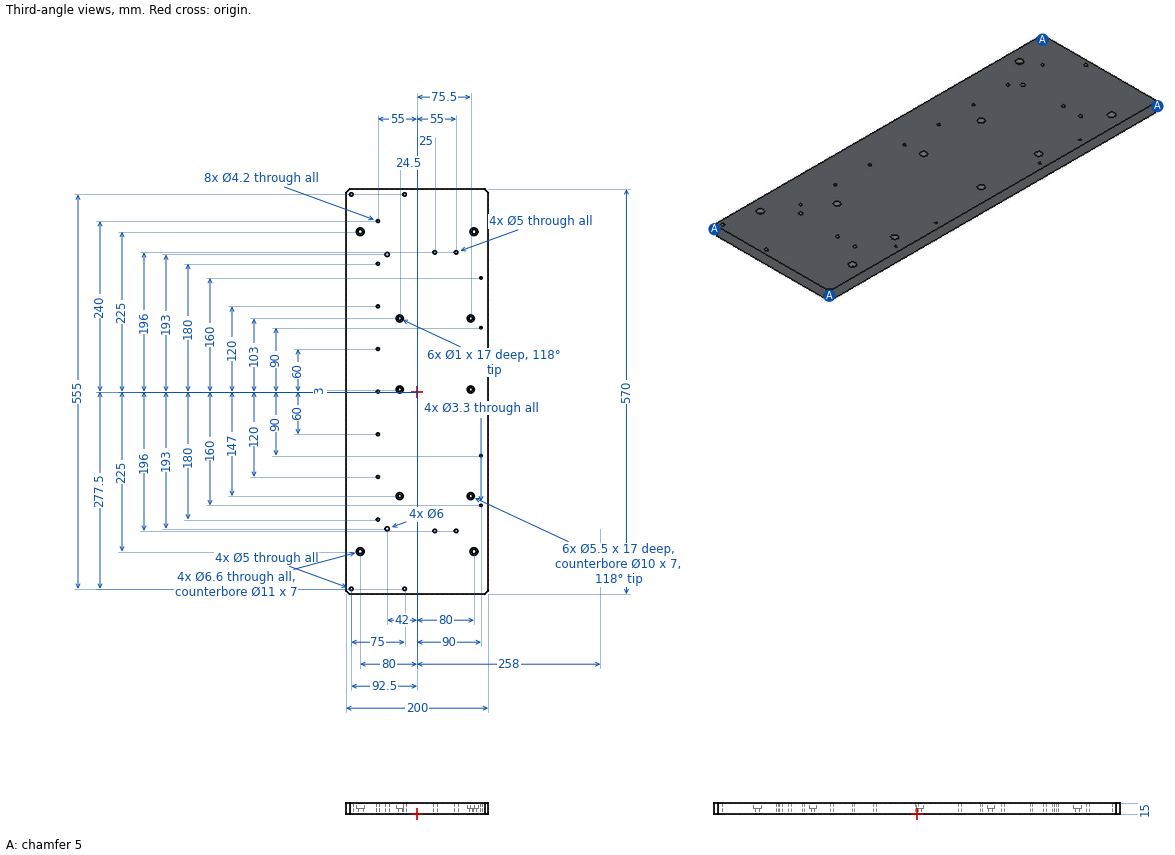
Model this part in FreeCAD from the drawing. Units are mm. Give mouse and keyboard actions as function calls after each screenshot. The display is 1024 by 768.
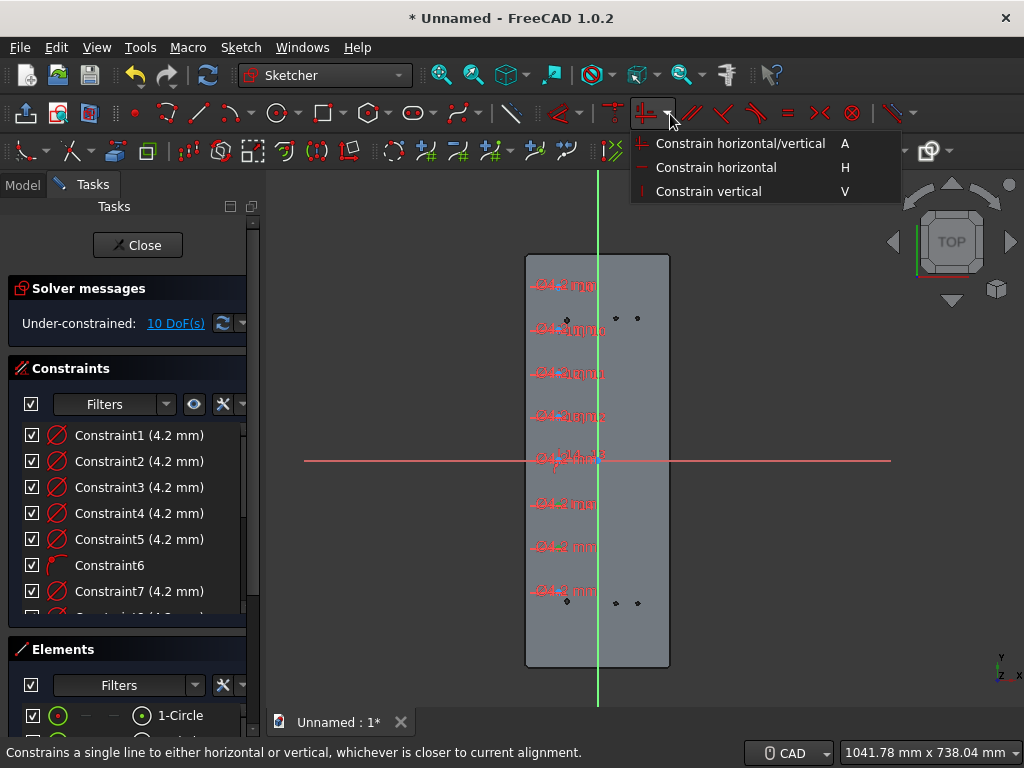
click(766, 191)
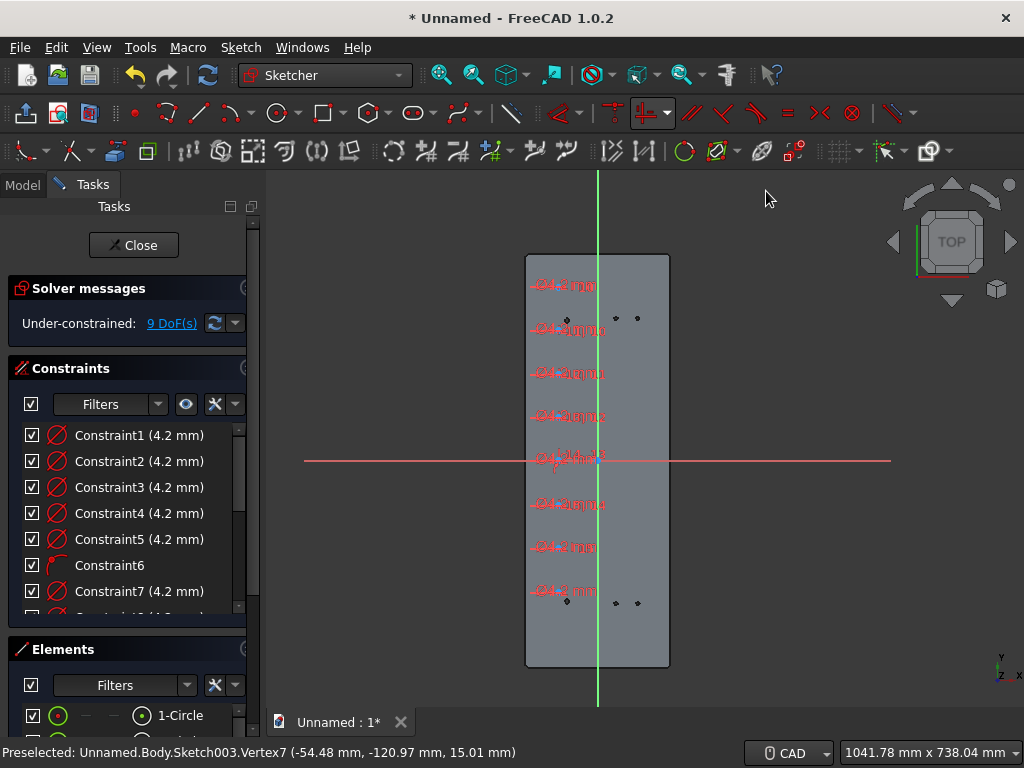
click(558, 549)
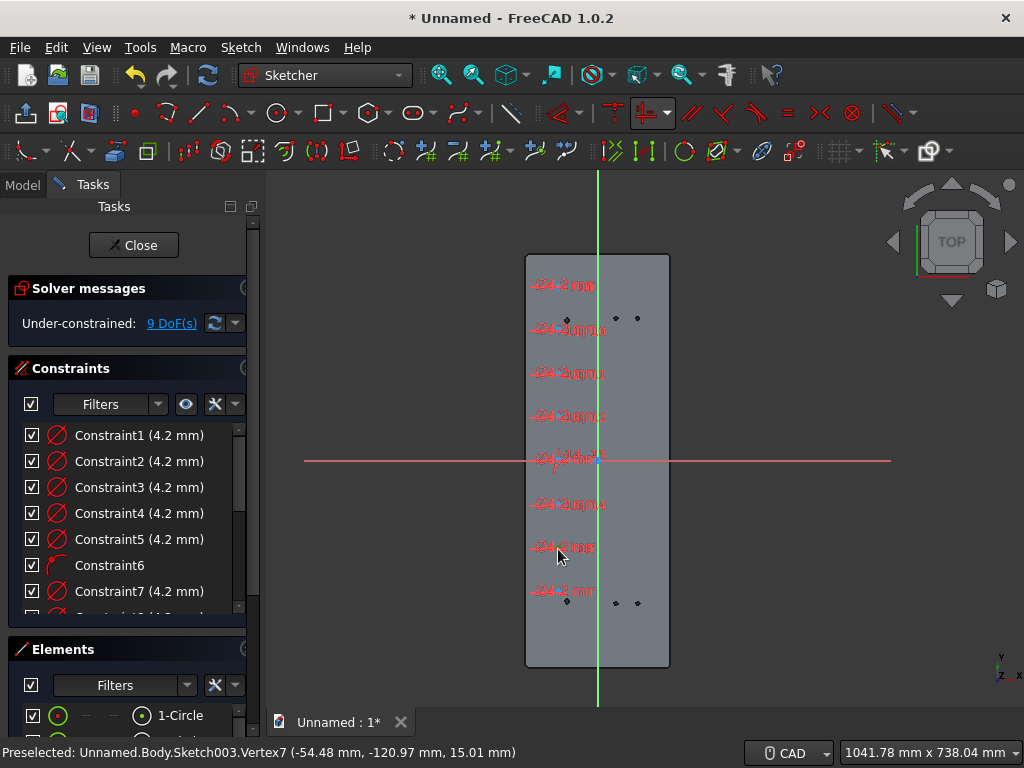
click(558, 593)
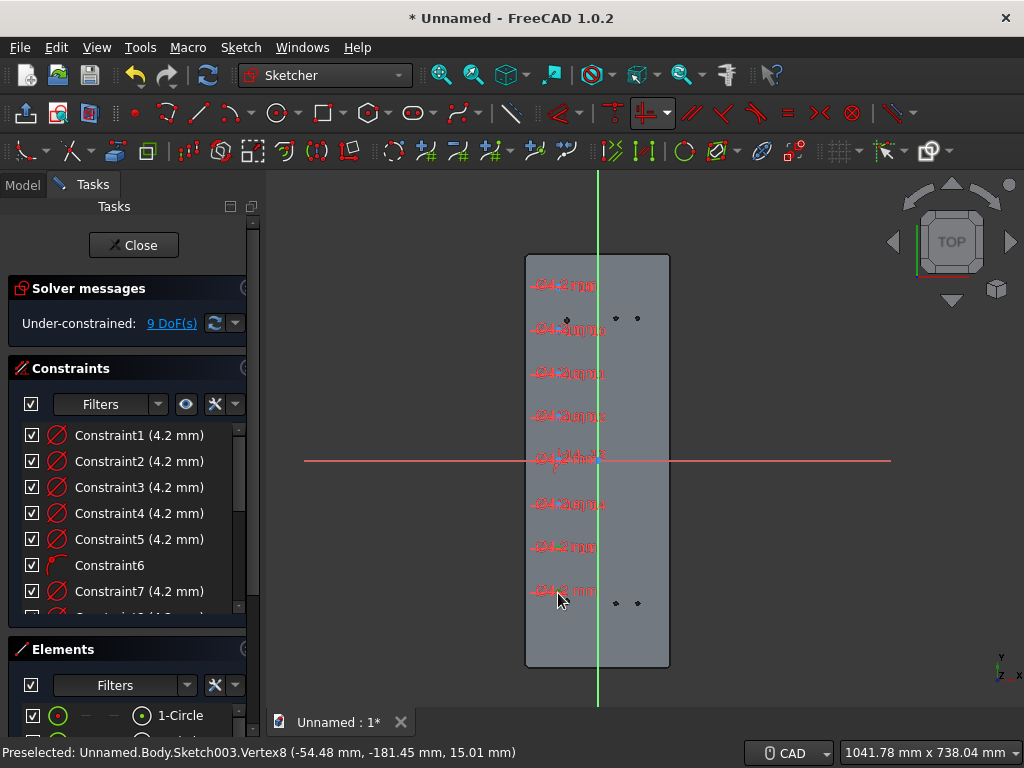
key(v)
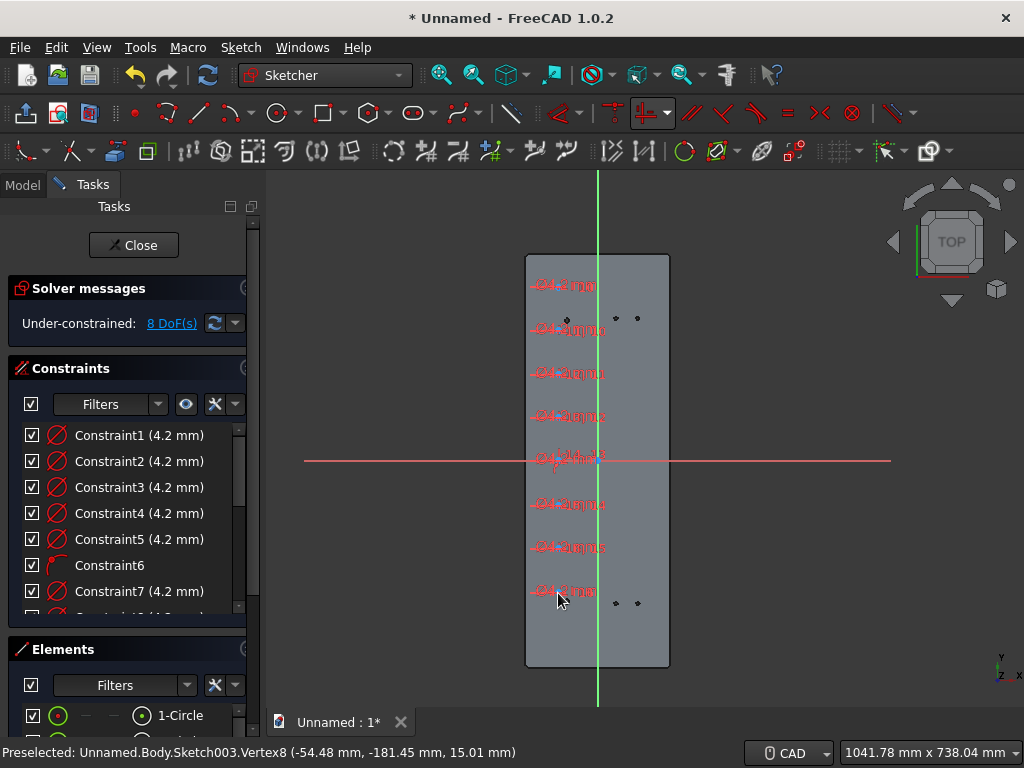
click(558, 114)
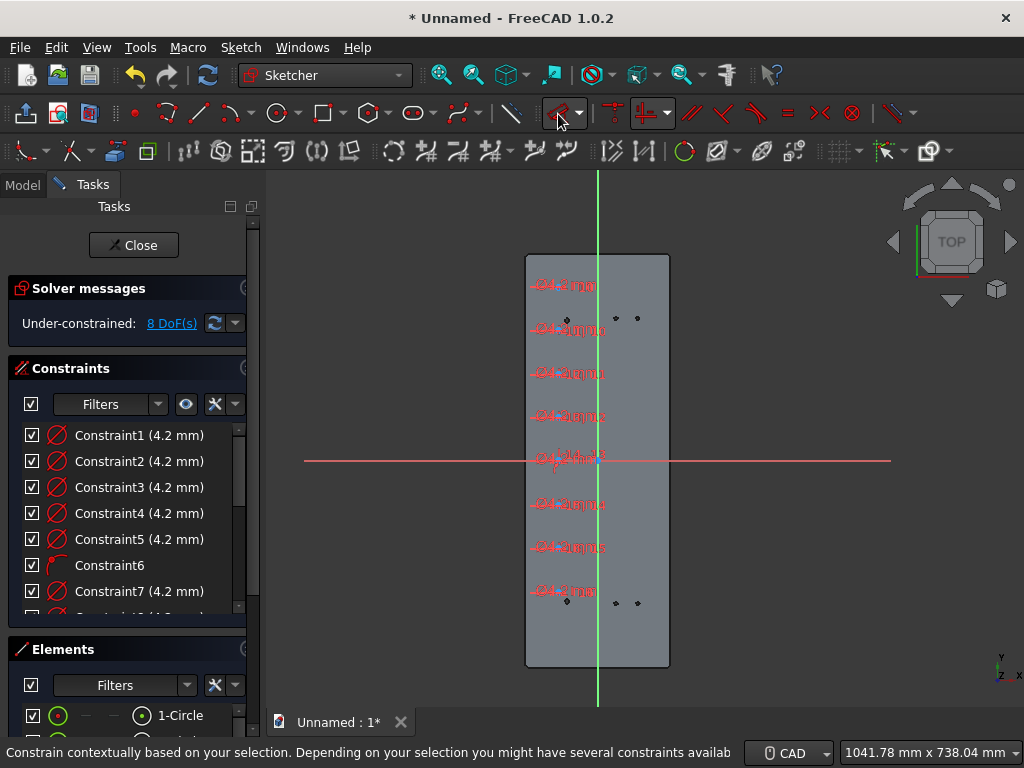
click(558, 287)
click(578, 253)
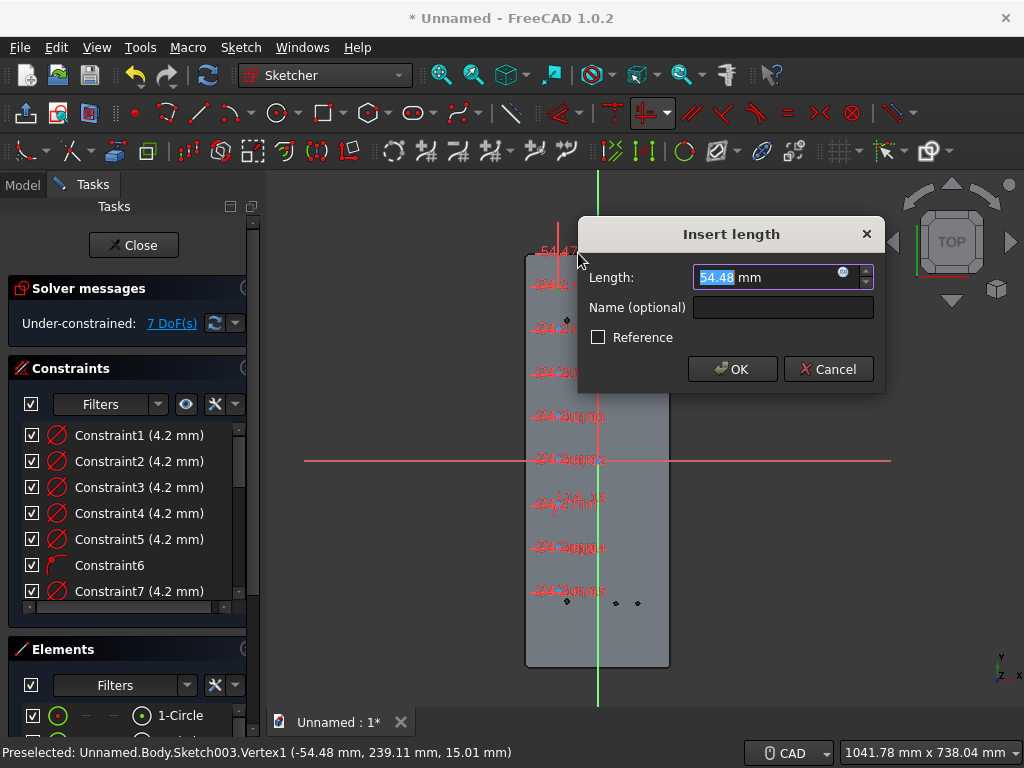
text(55)
key(Return)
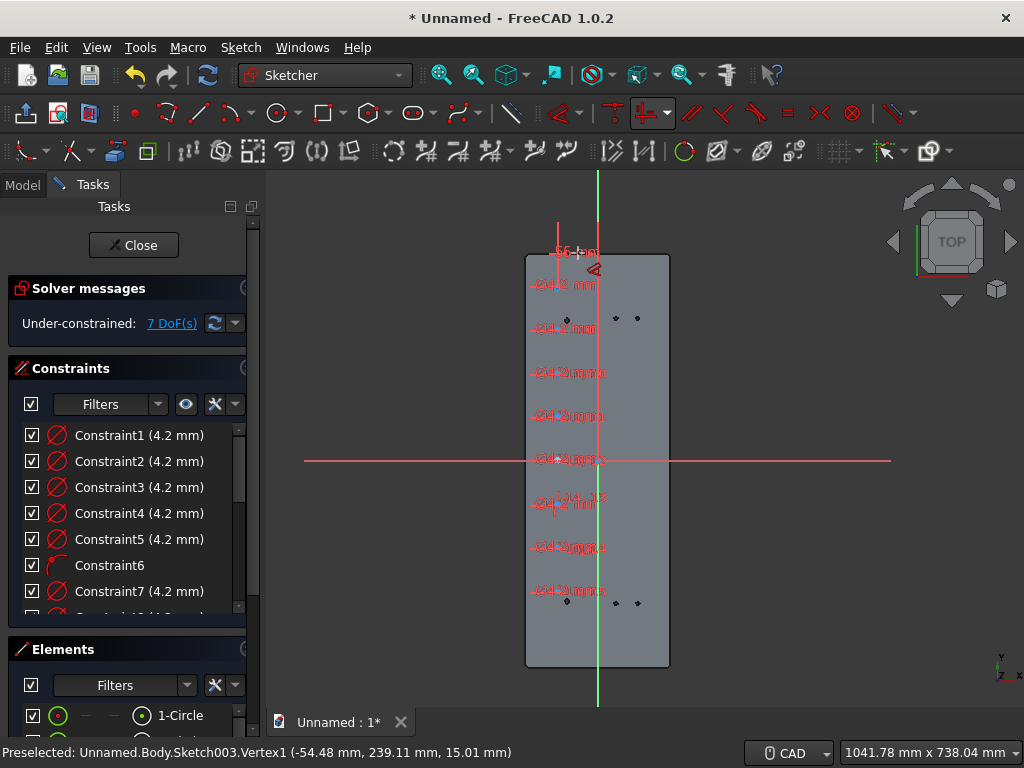
click(558, 418)
click(632, 439)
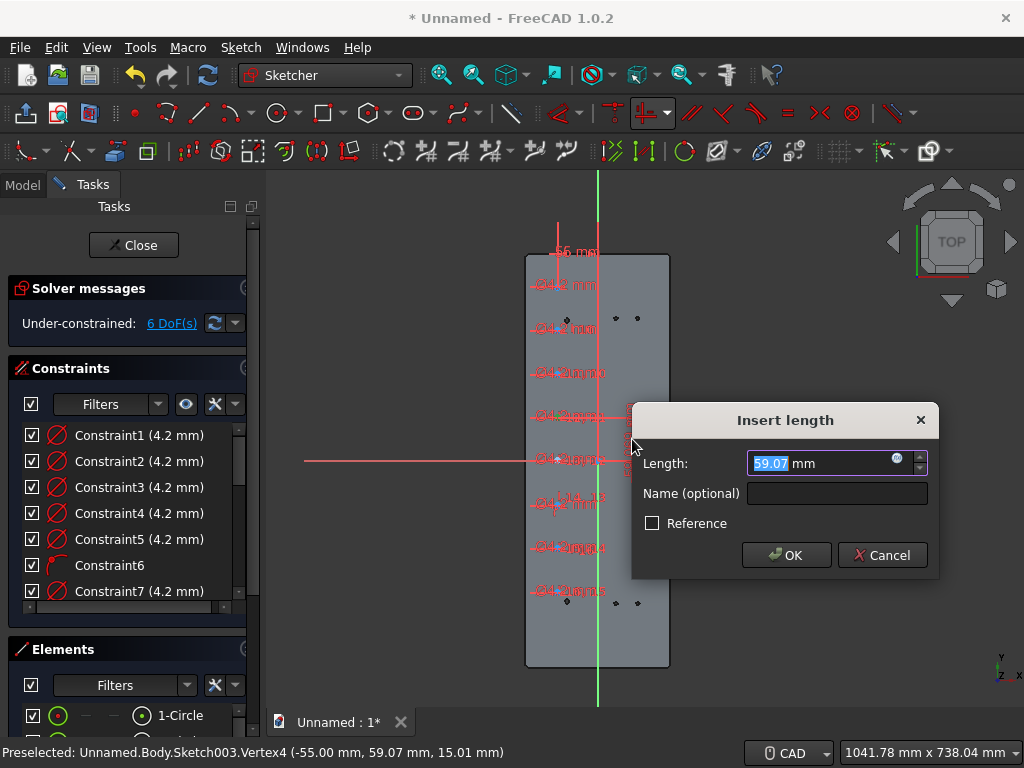
text(60)
key(Return)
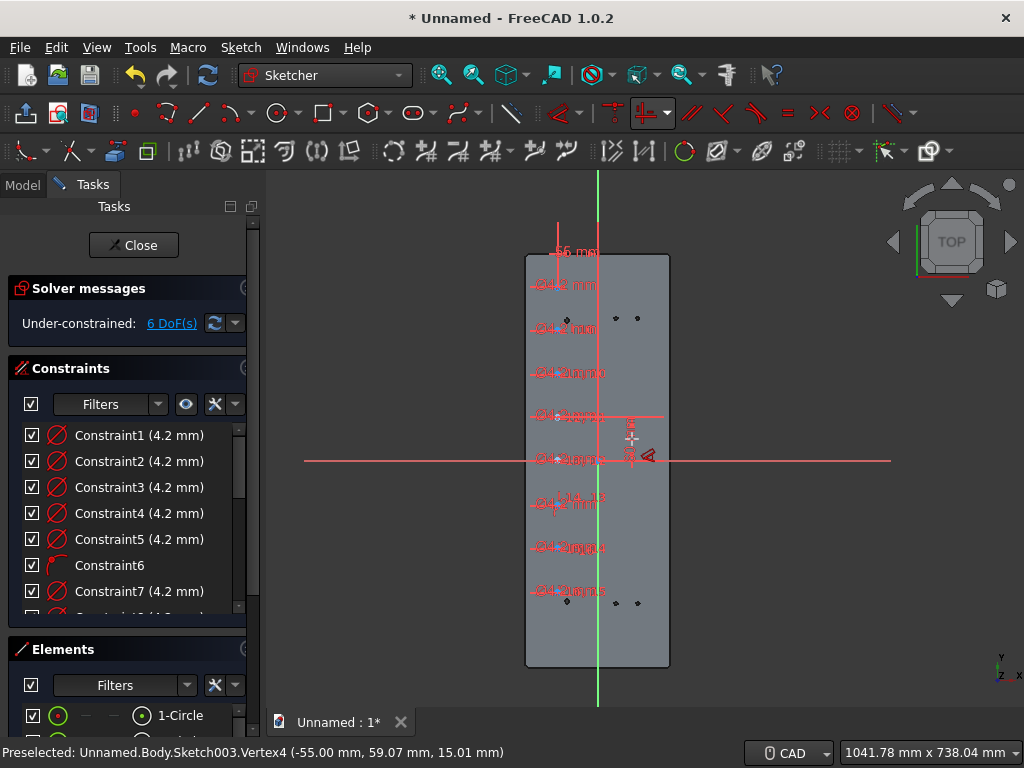
click(558, 506)
click(632, 483)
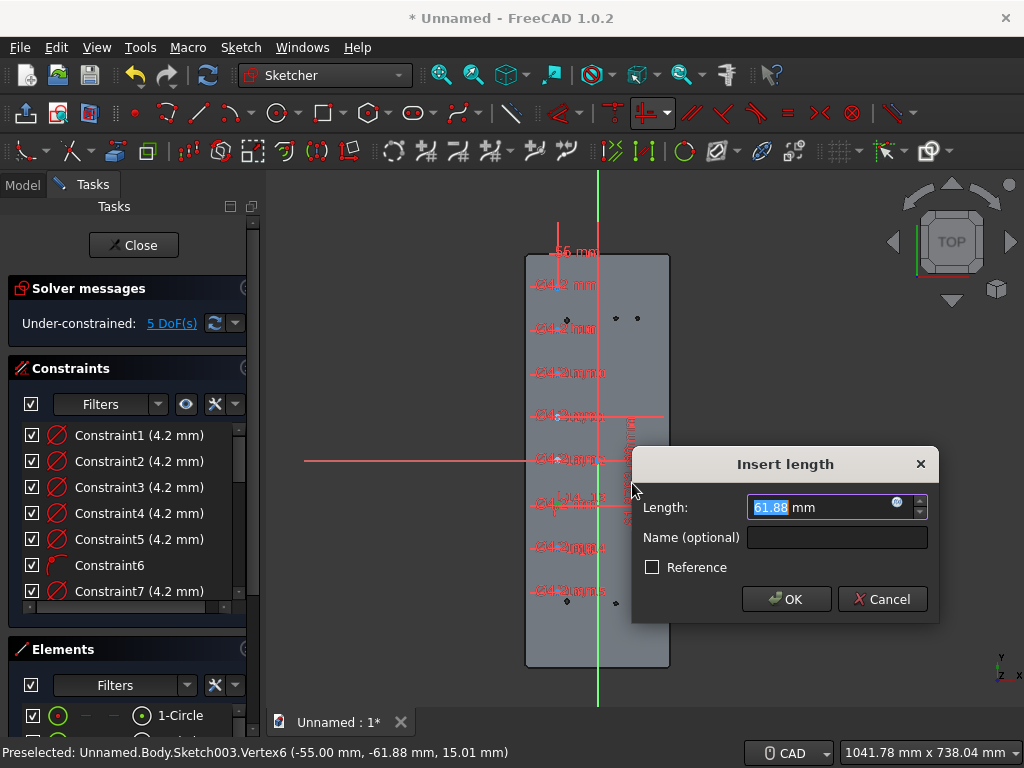
text(60)
key(Return)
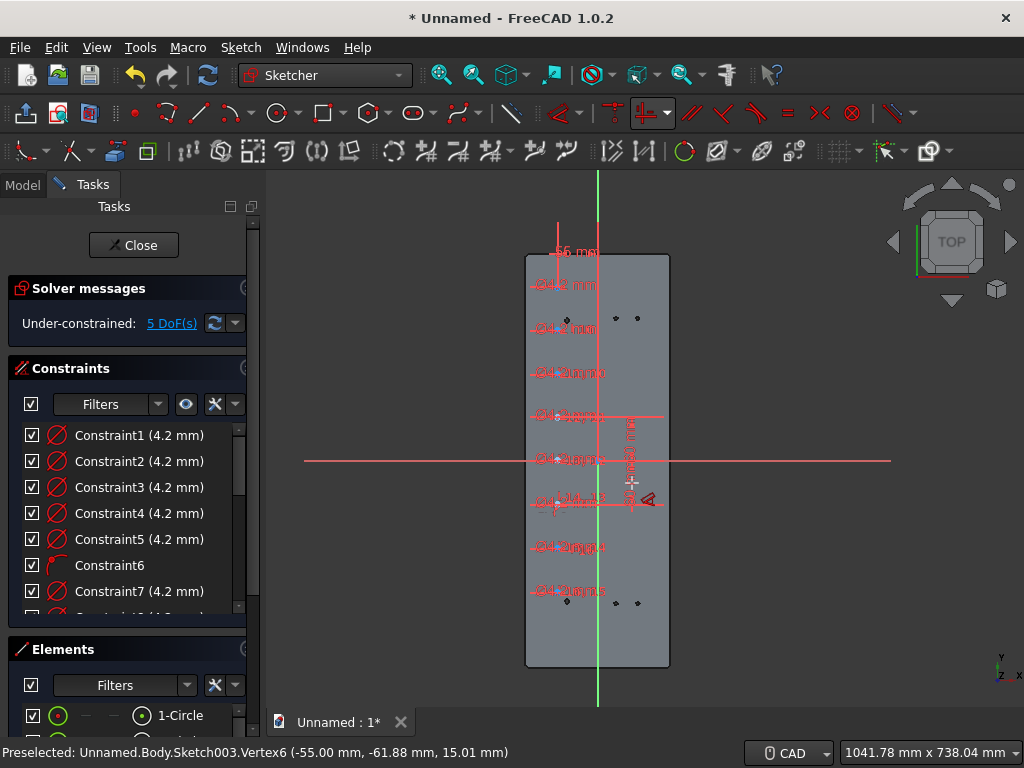
click(558, 287)
click(632, 374)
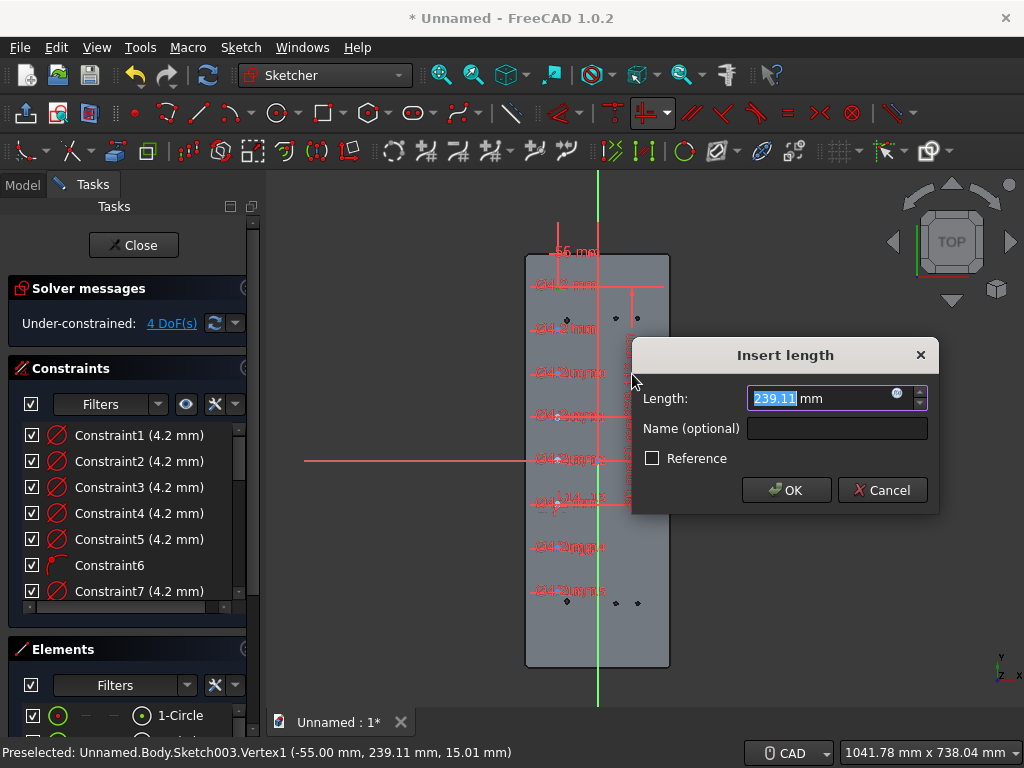
text(240)
key(Return)